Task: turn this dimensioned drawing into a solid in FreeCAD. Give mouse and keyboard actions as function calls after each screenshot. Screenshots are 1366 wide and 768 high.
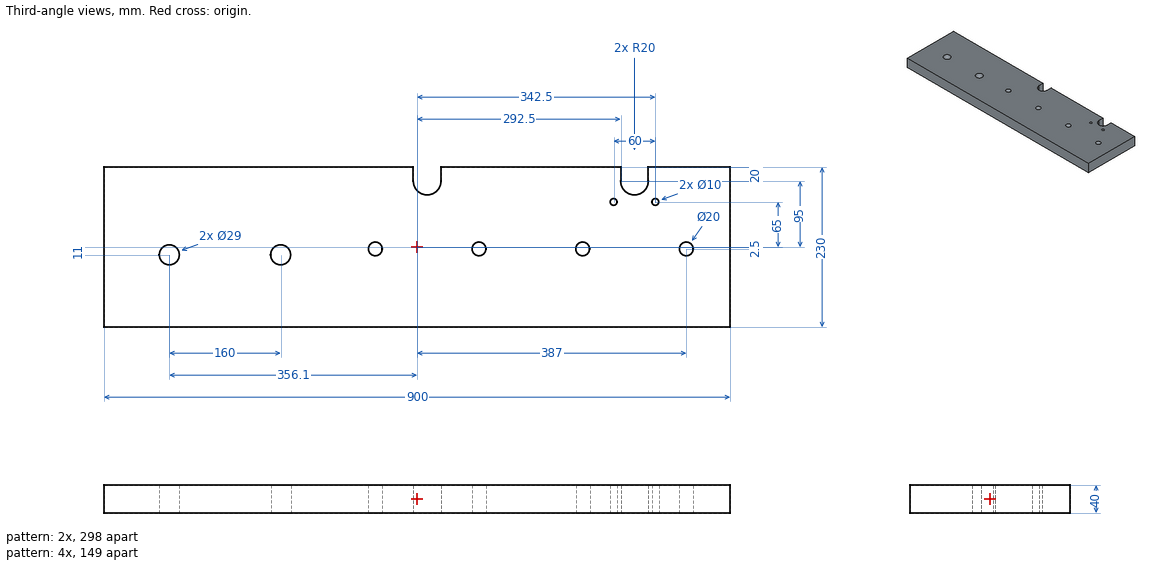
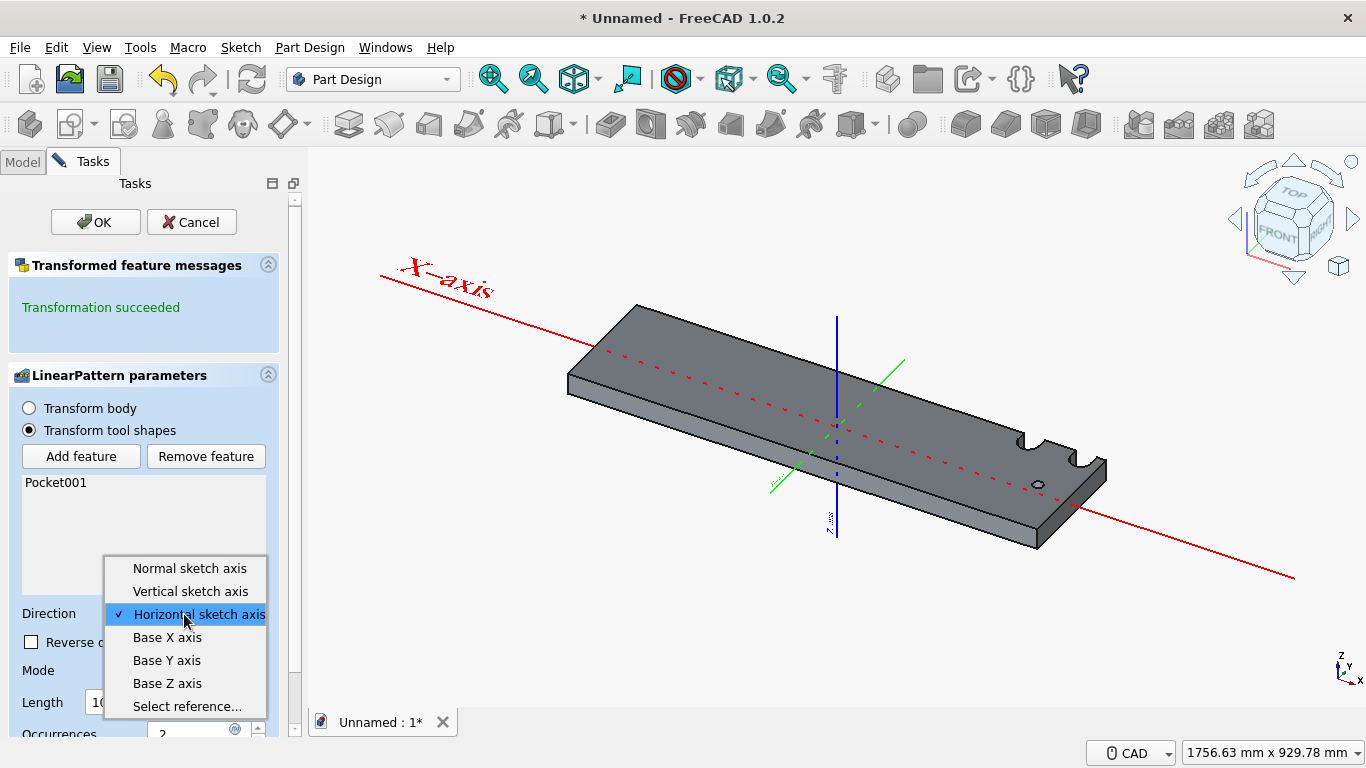
click(184, 638)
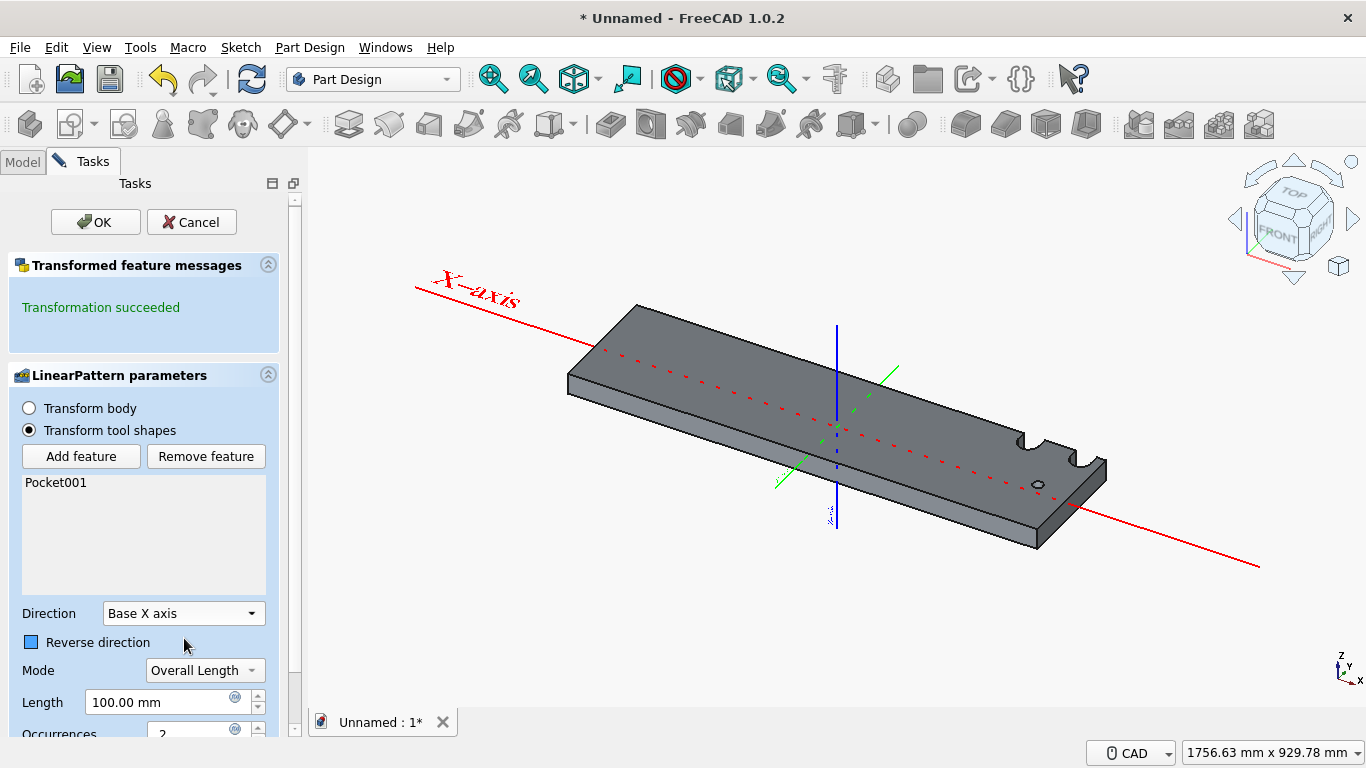
click(206, 670)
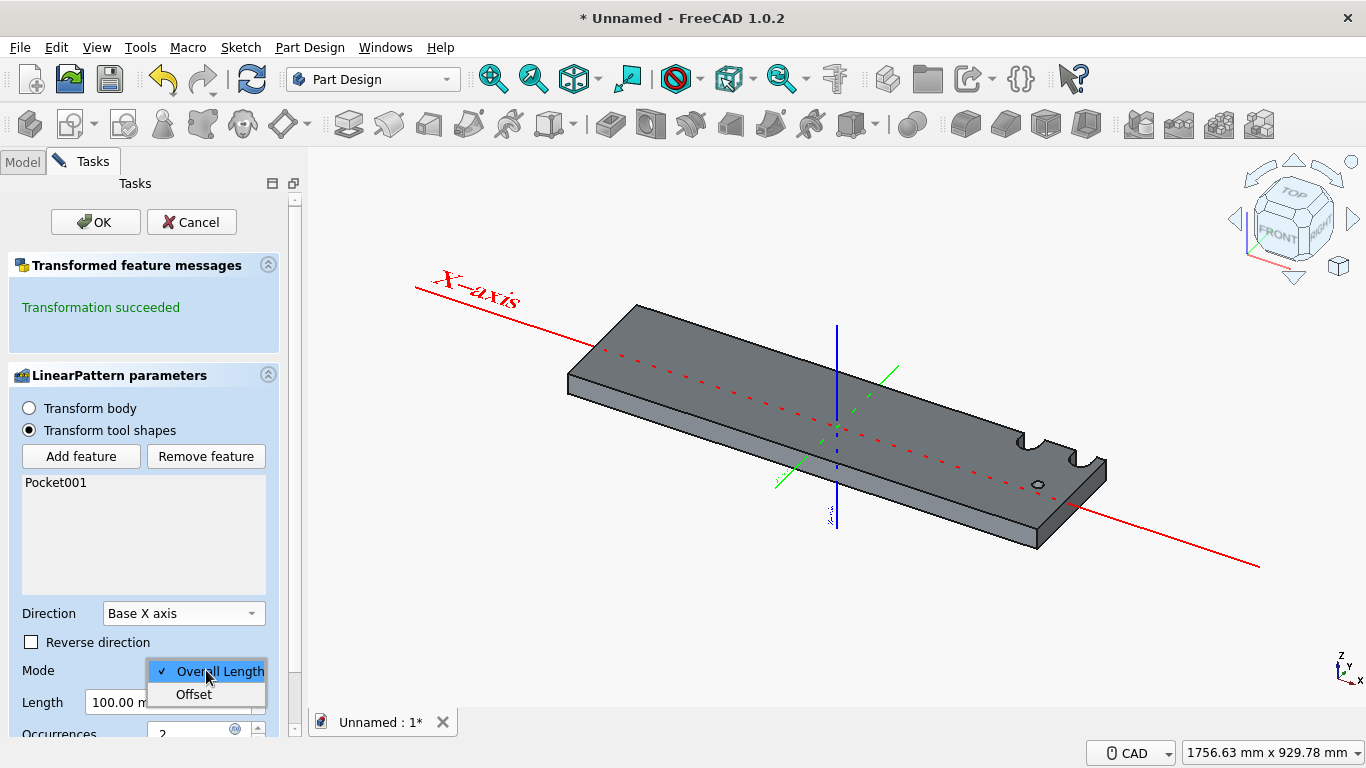
click(206, 694)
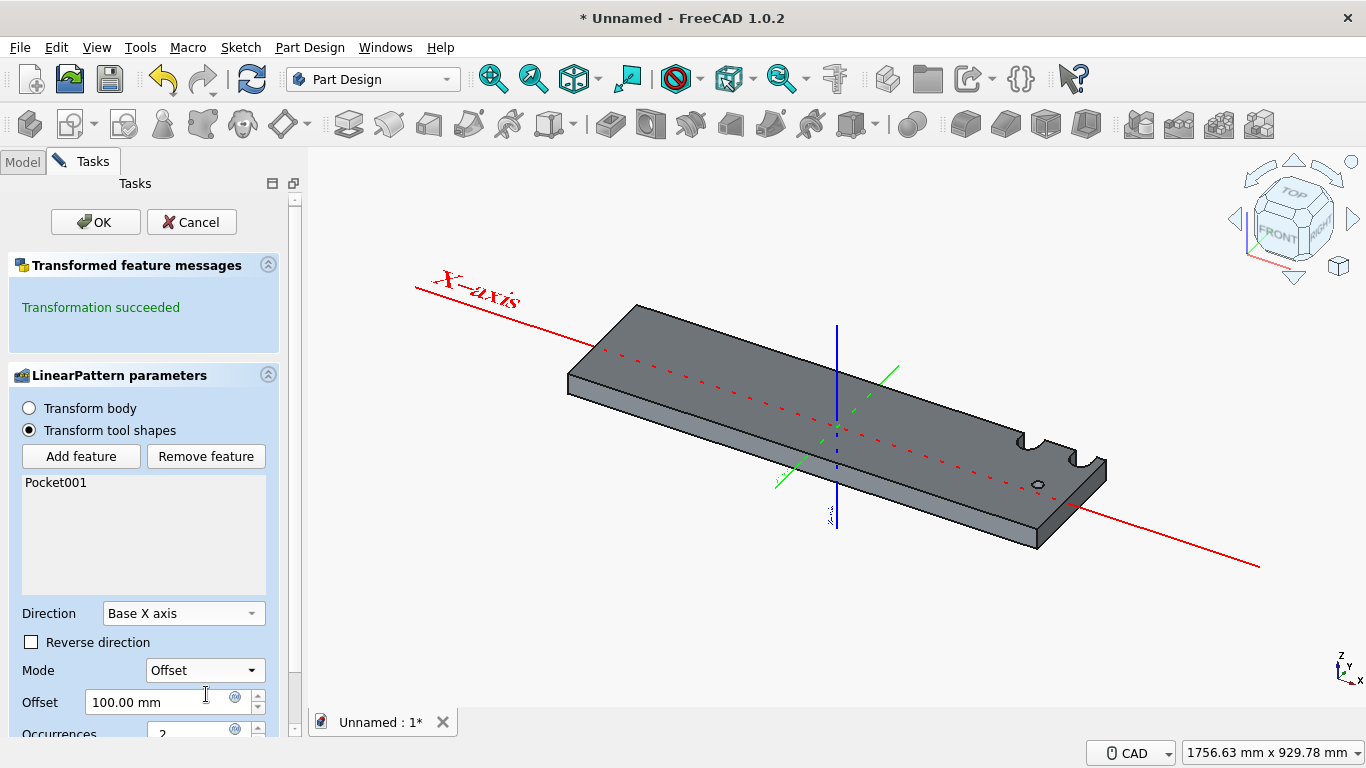
triple_click(168, 702)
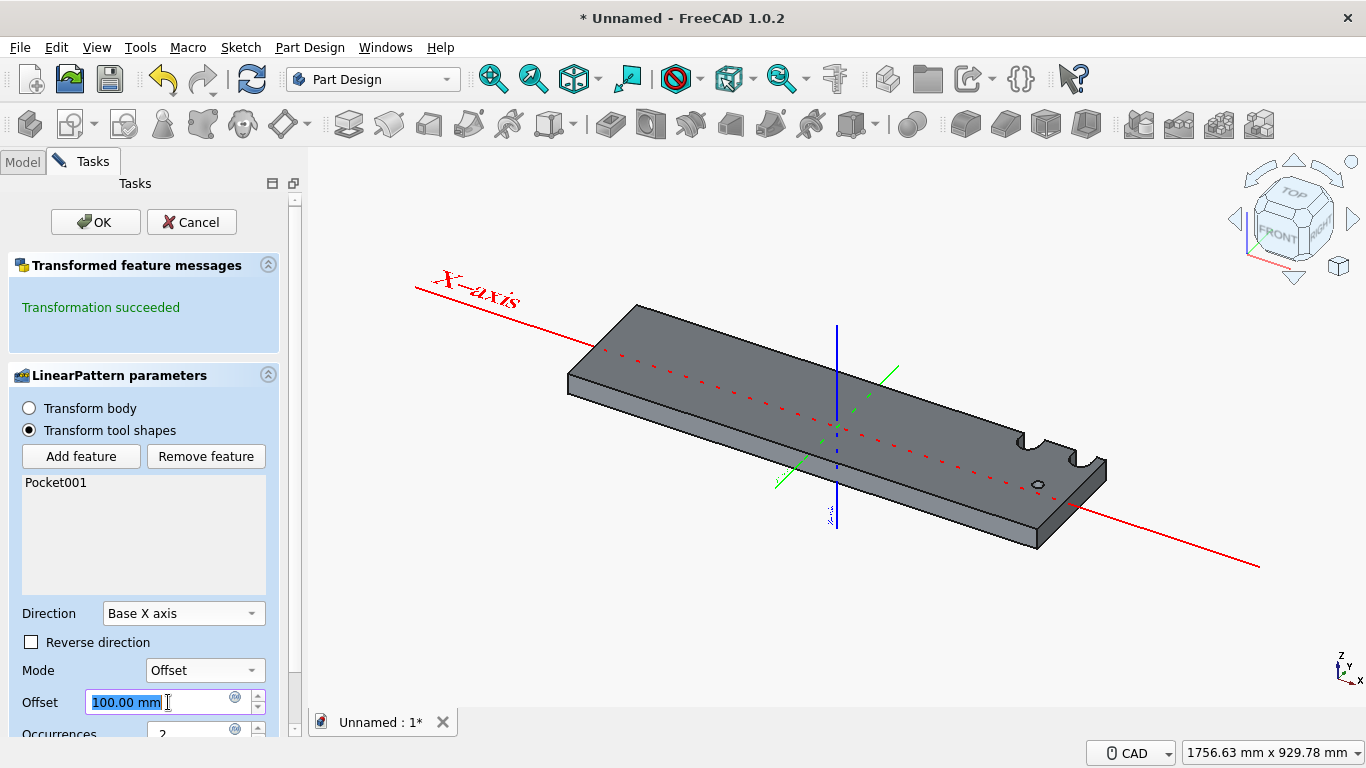
text(298)
key(Tab)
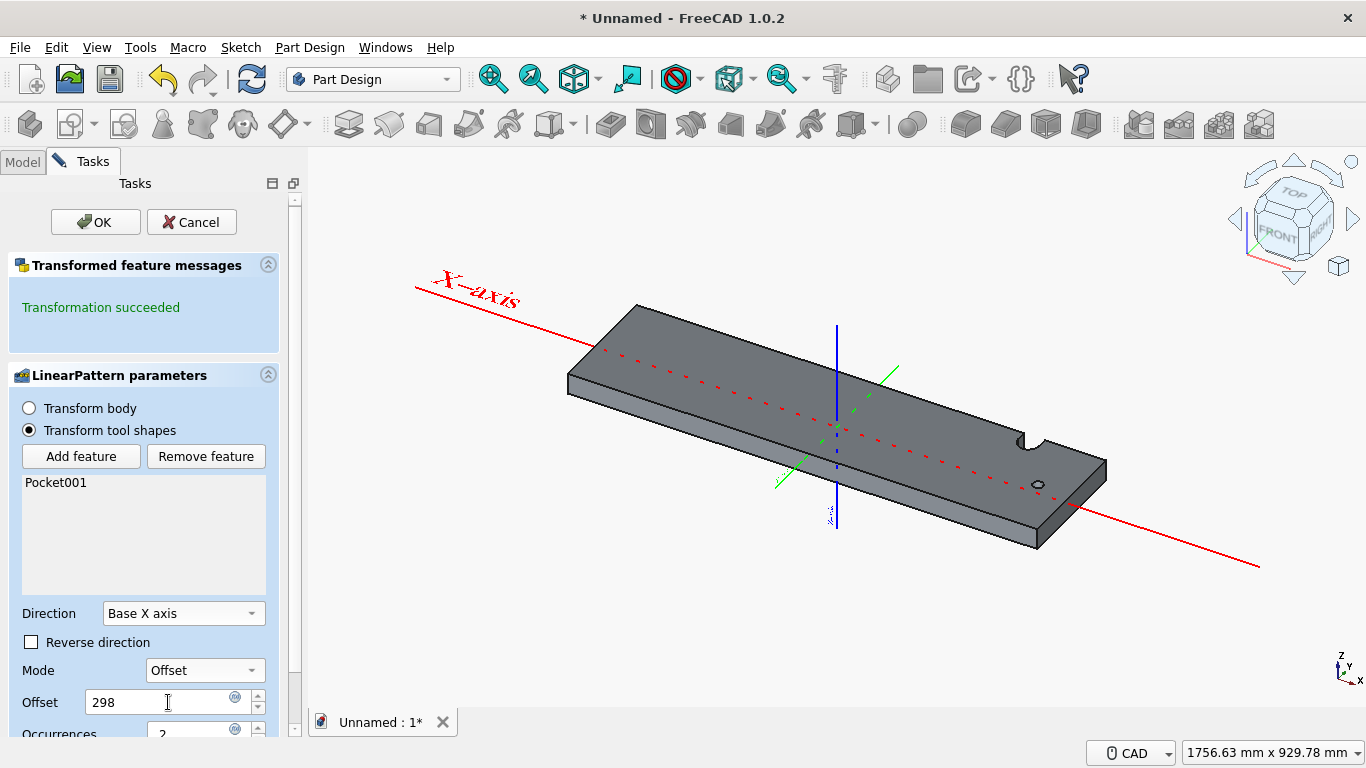
scroll(295, 464, down, 2)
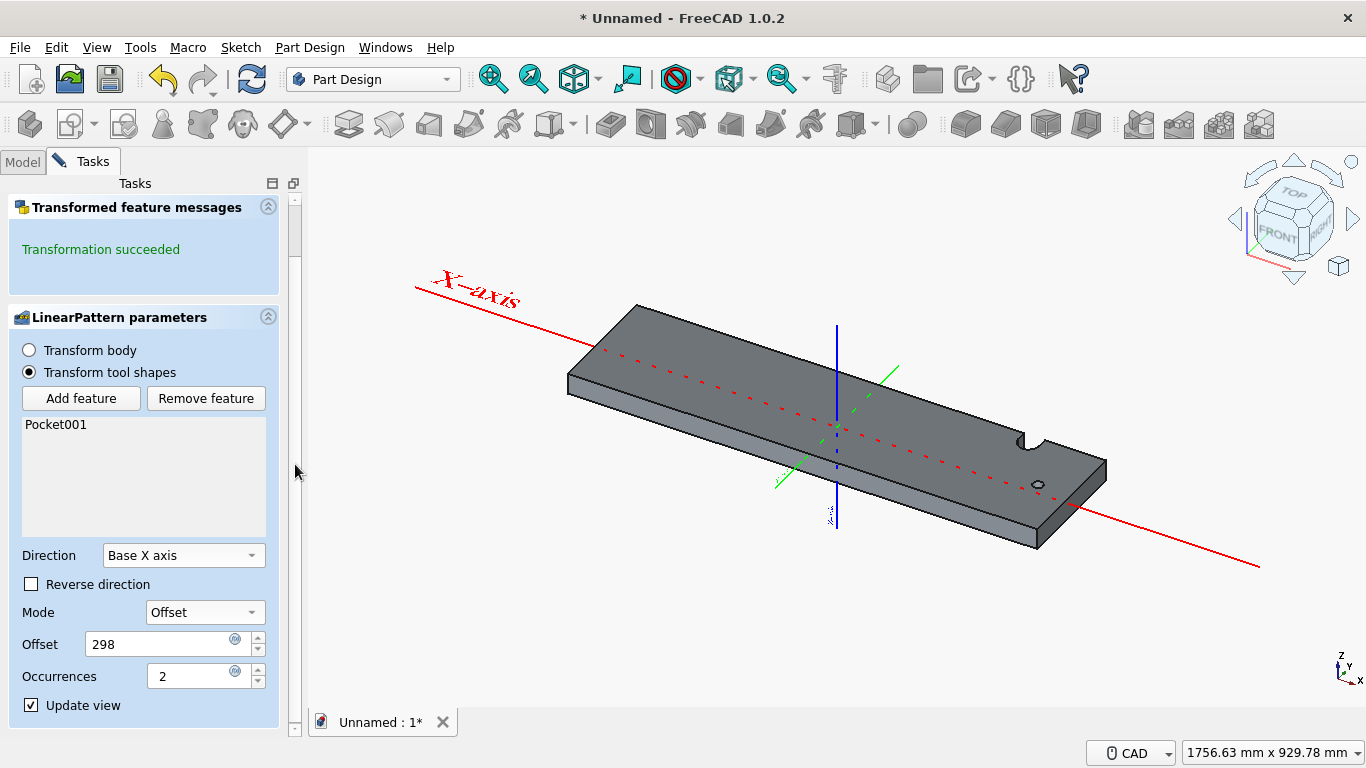
triple_click(198, 676)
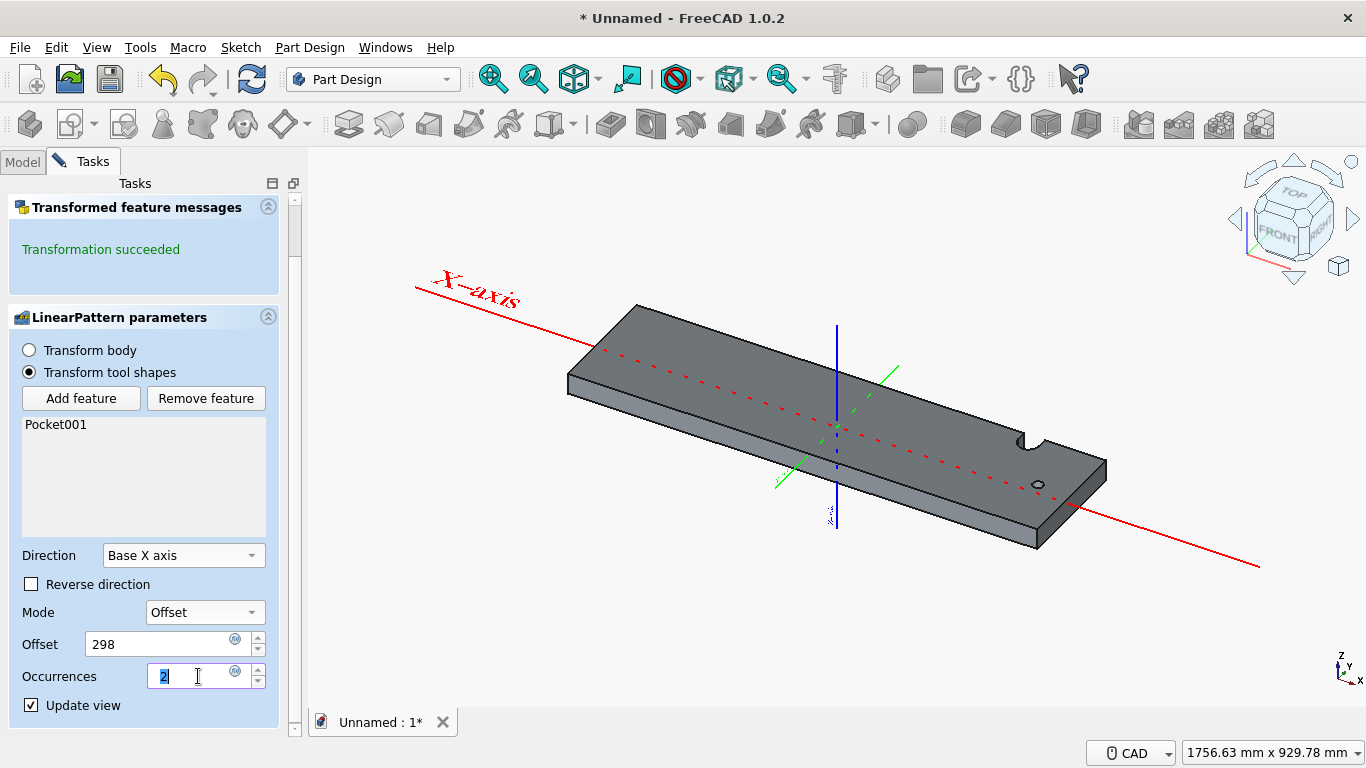
text(2)
key(Tab)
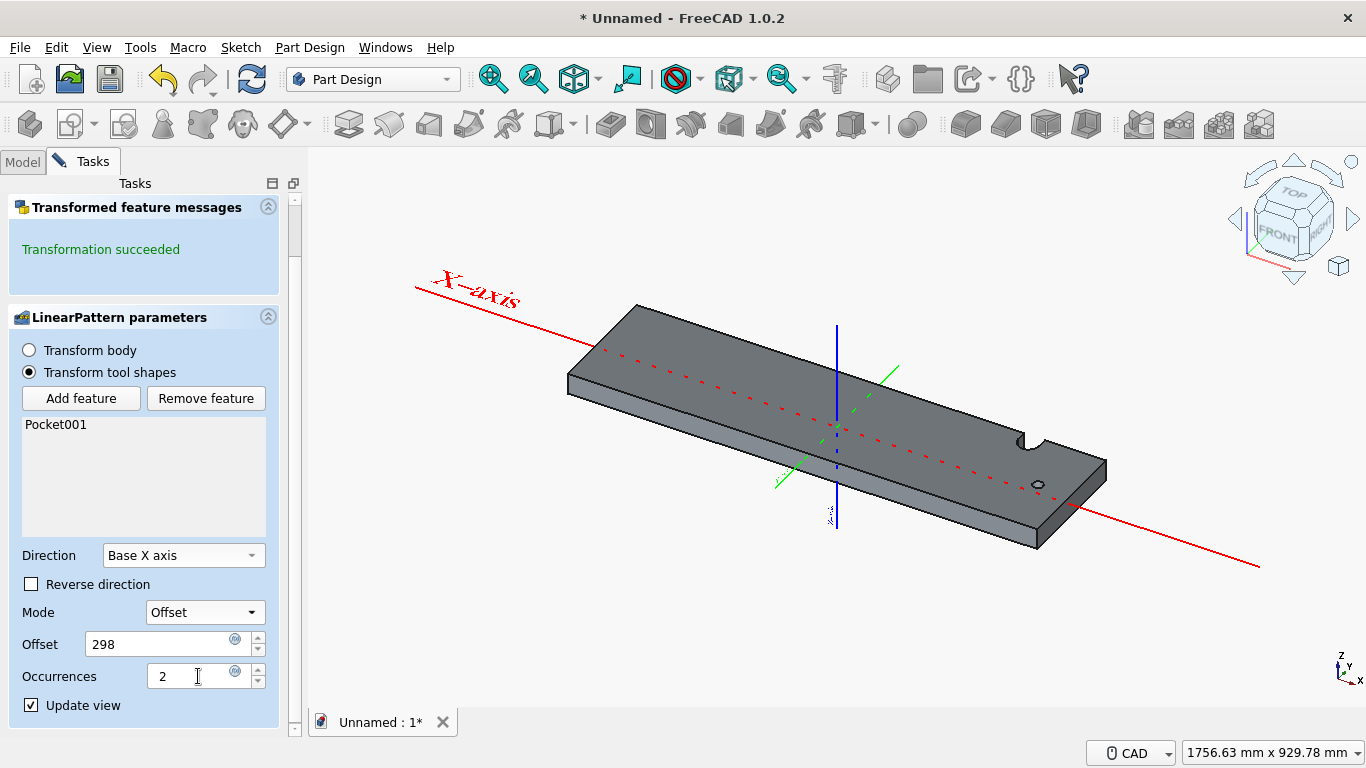
click(30, 584)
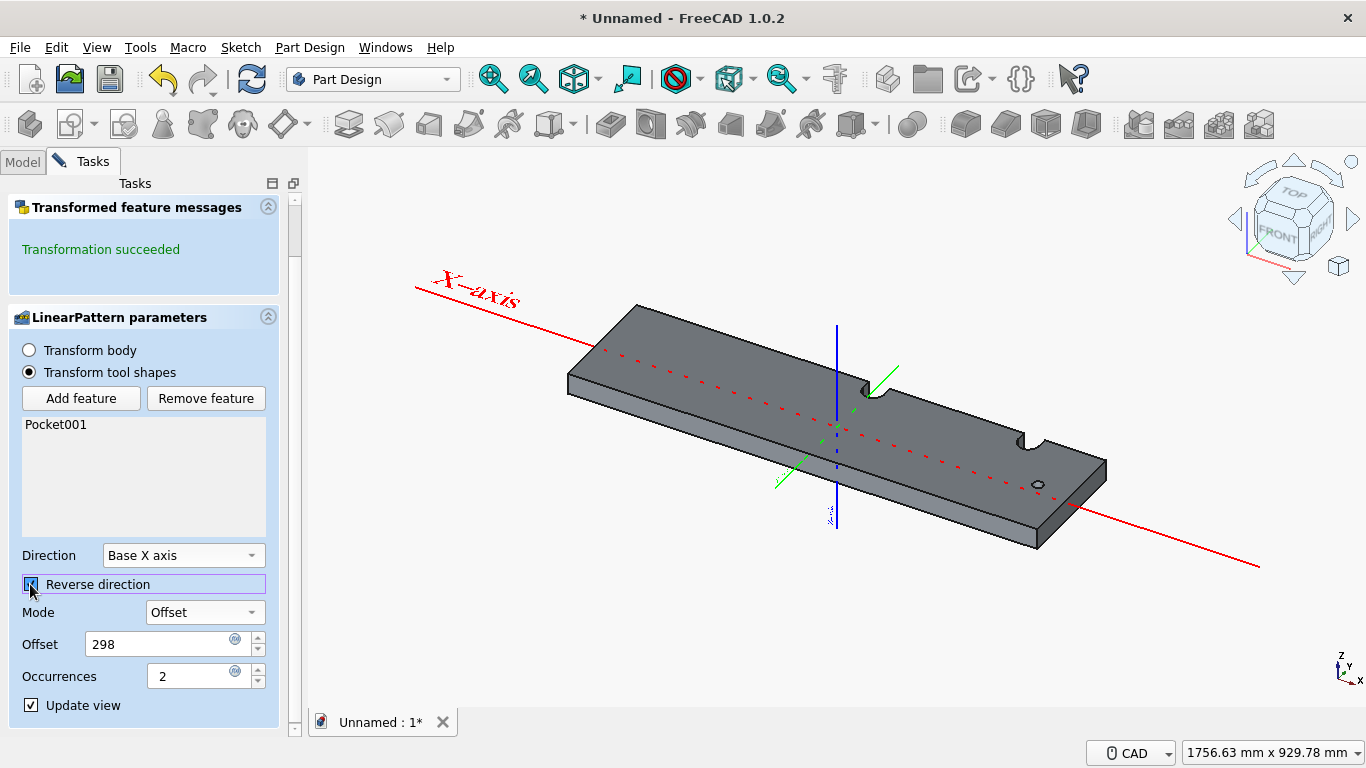
scroll(295, 464, up, 2)